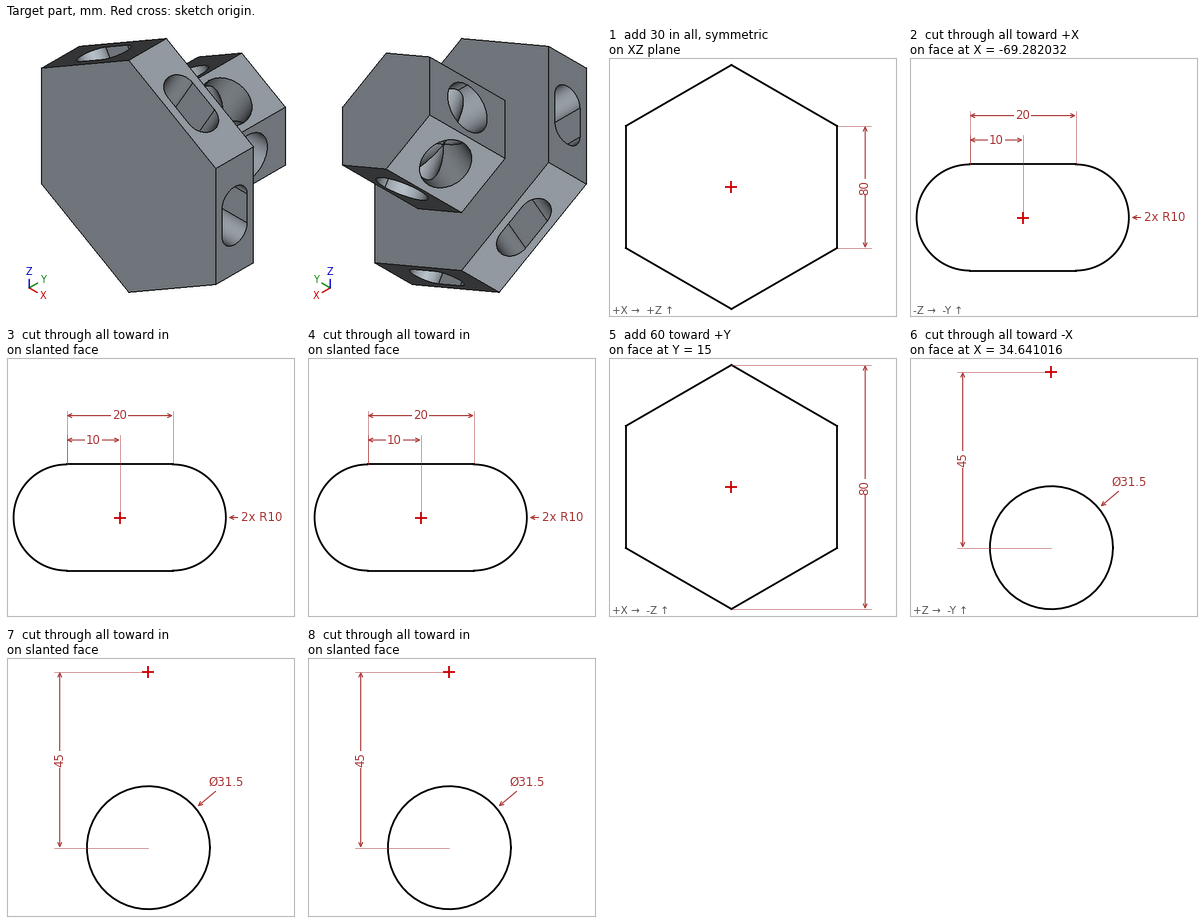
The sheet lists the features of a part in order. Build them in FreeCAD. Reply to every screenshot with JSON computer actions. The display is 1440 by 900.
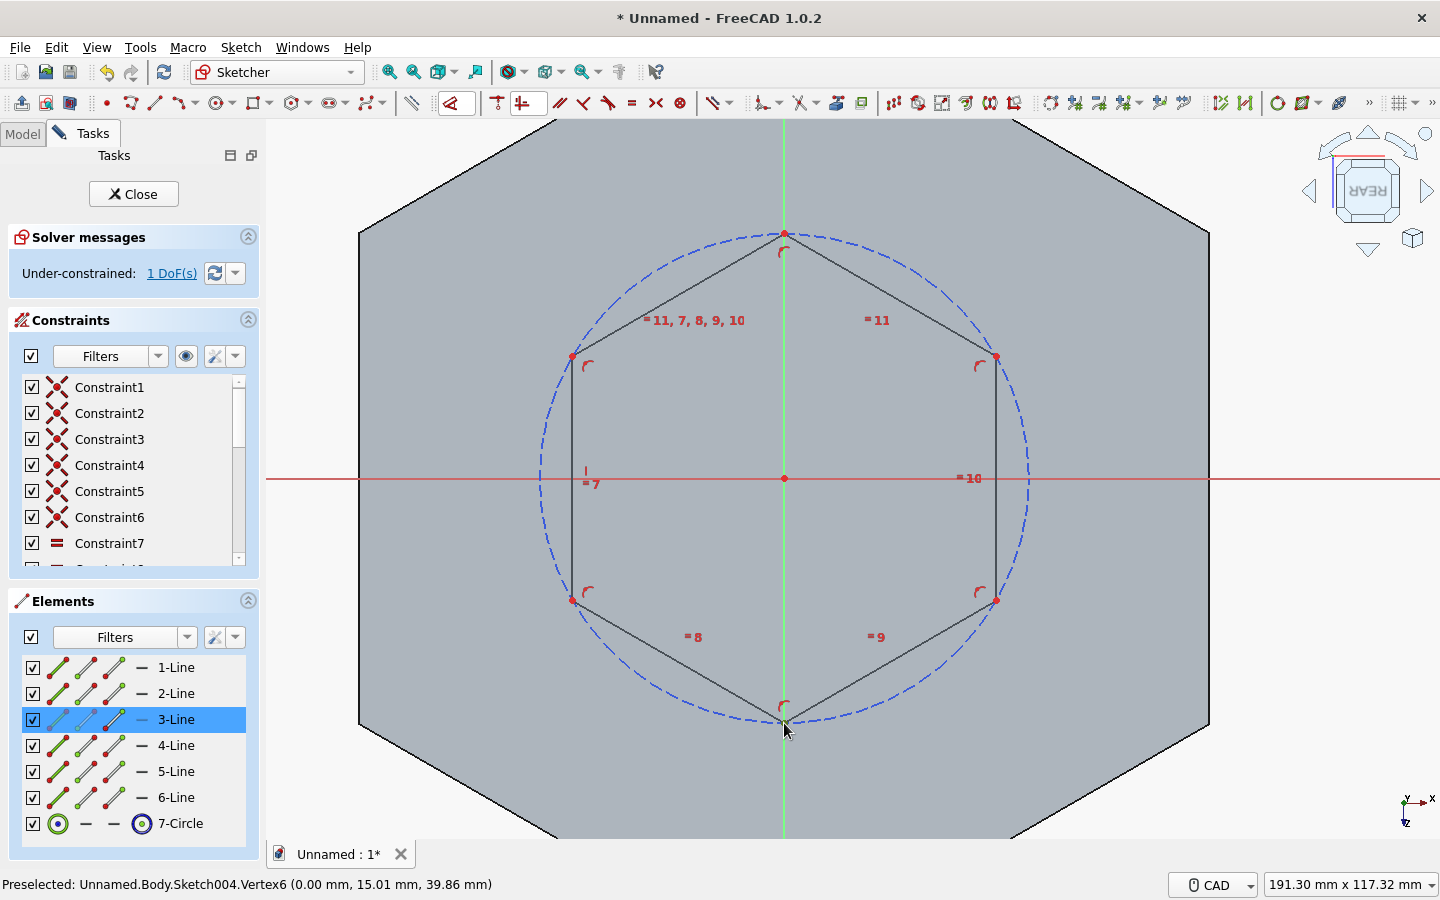
{"action": "left_click", "coordinate": [784, 234]}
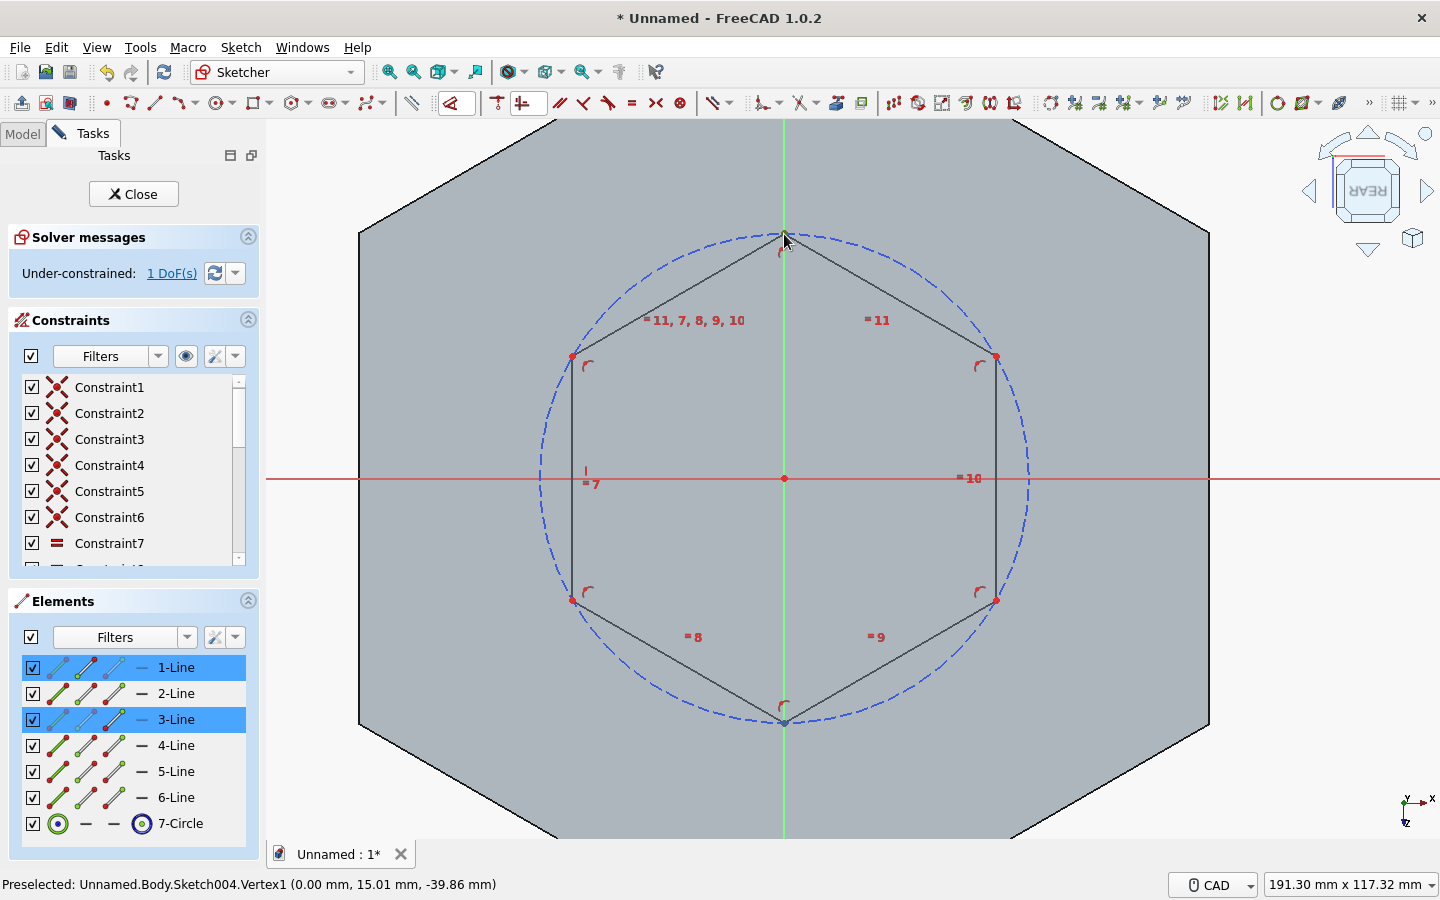
{"action": "key", "text": "i"}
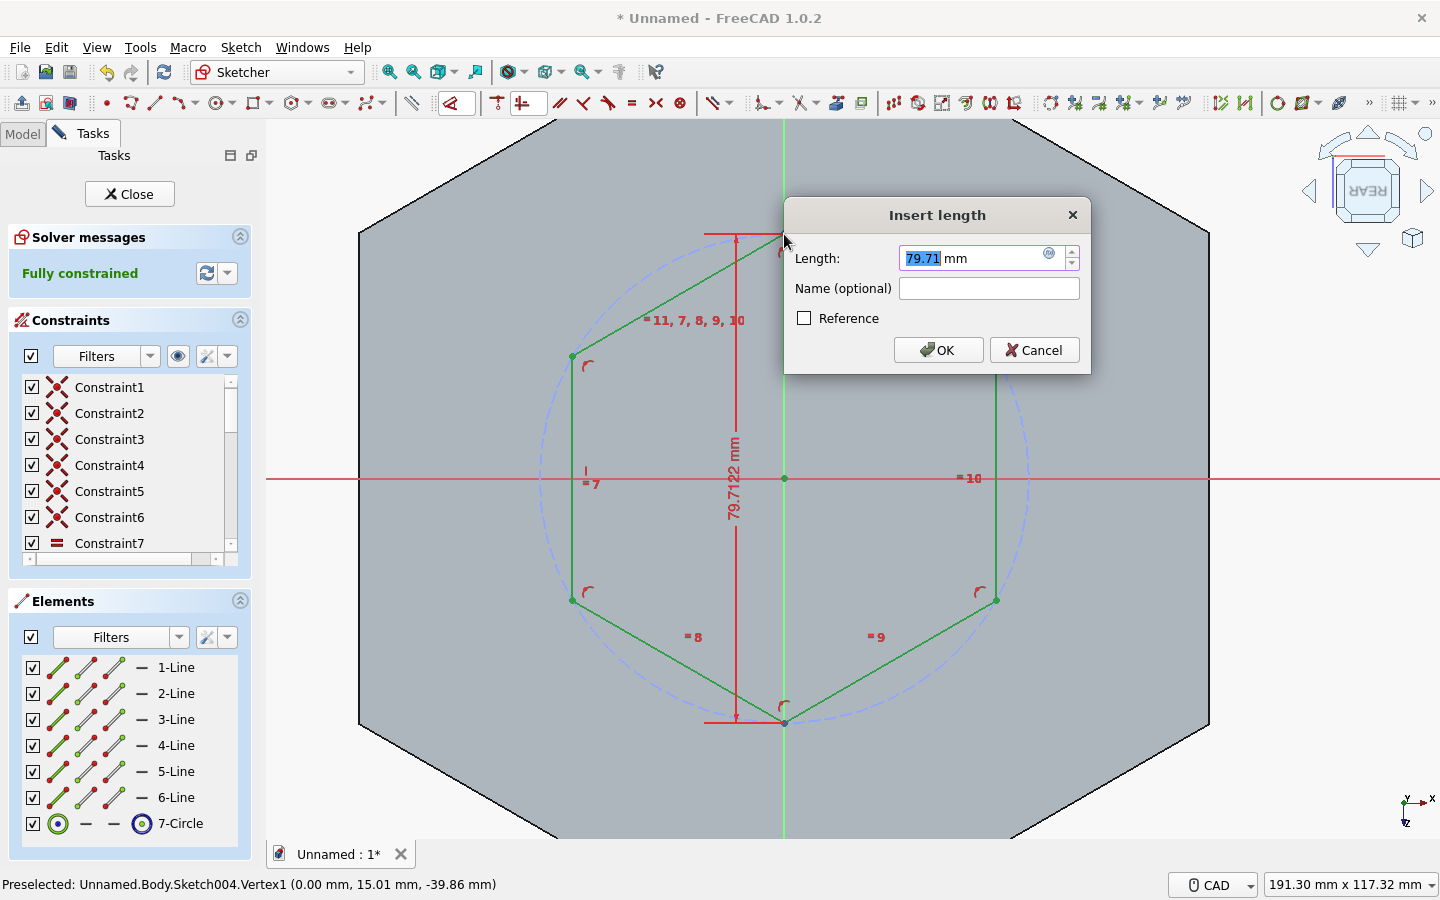
{"action": "type", "text": "80"}
{"action": "key", "text": "Return"}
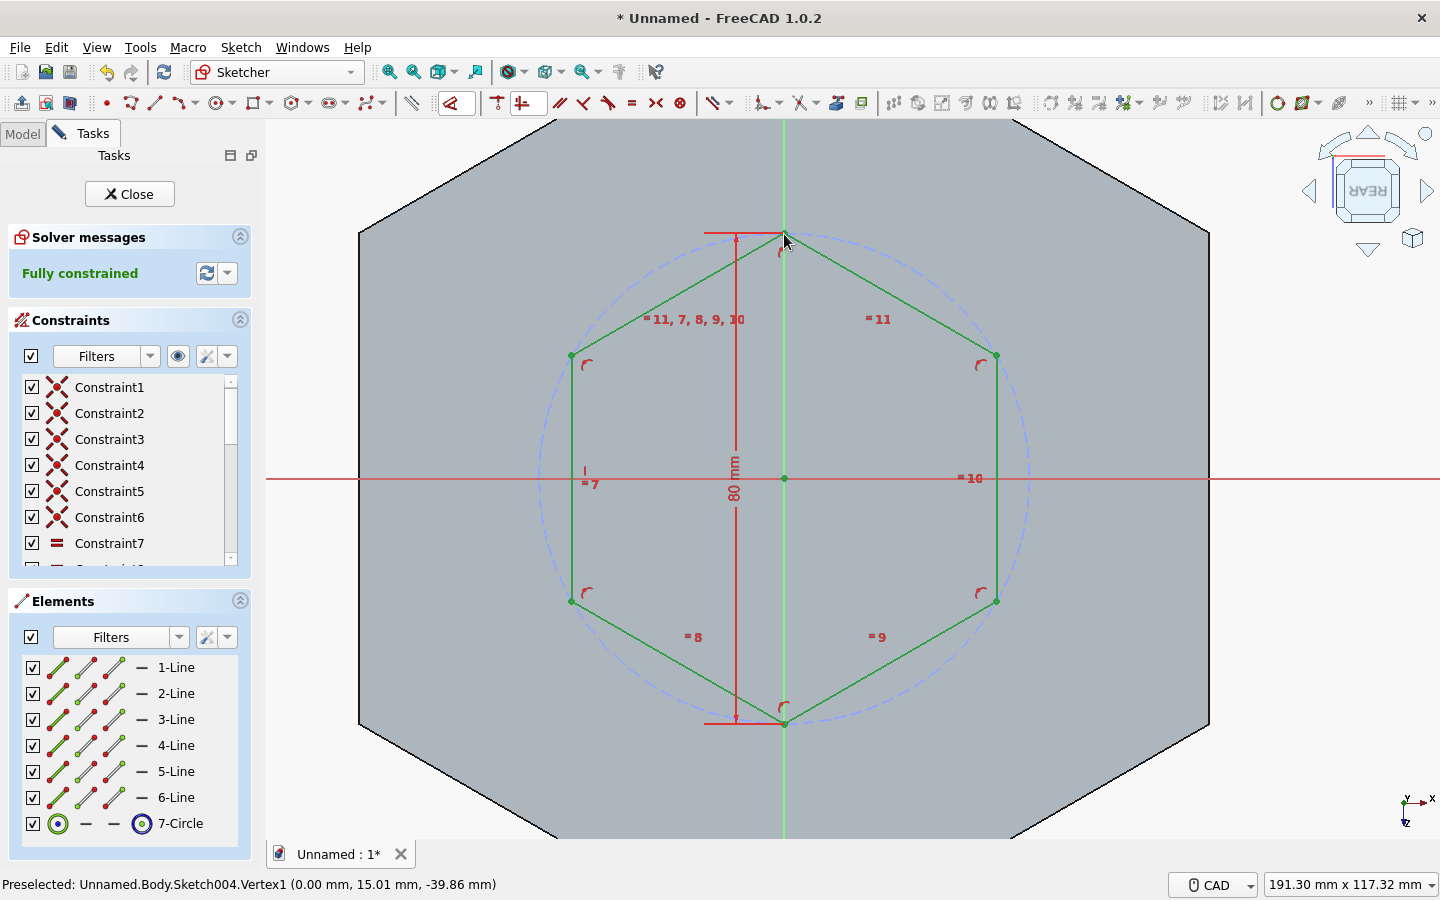
{"action": "left_click", "coordinate": [130, 194]}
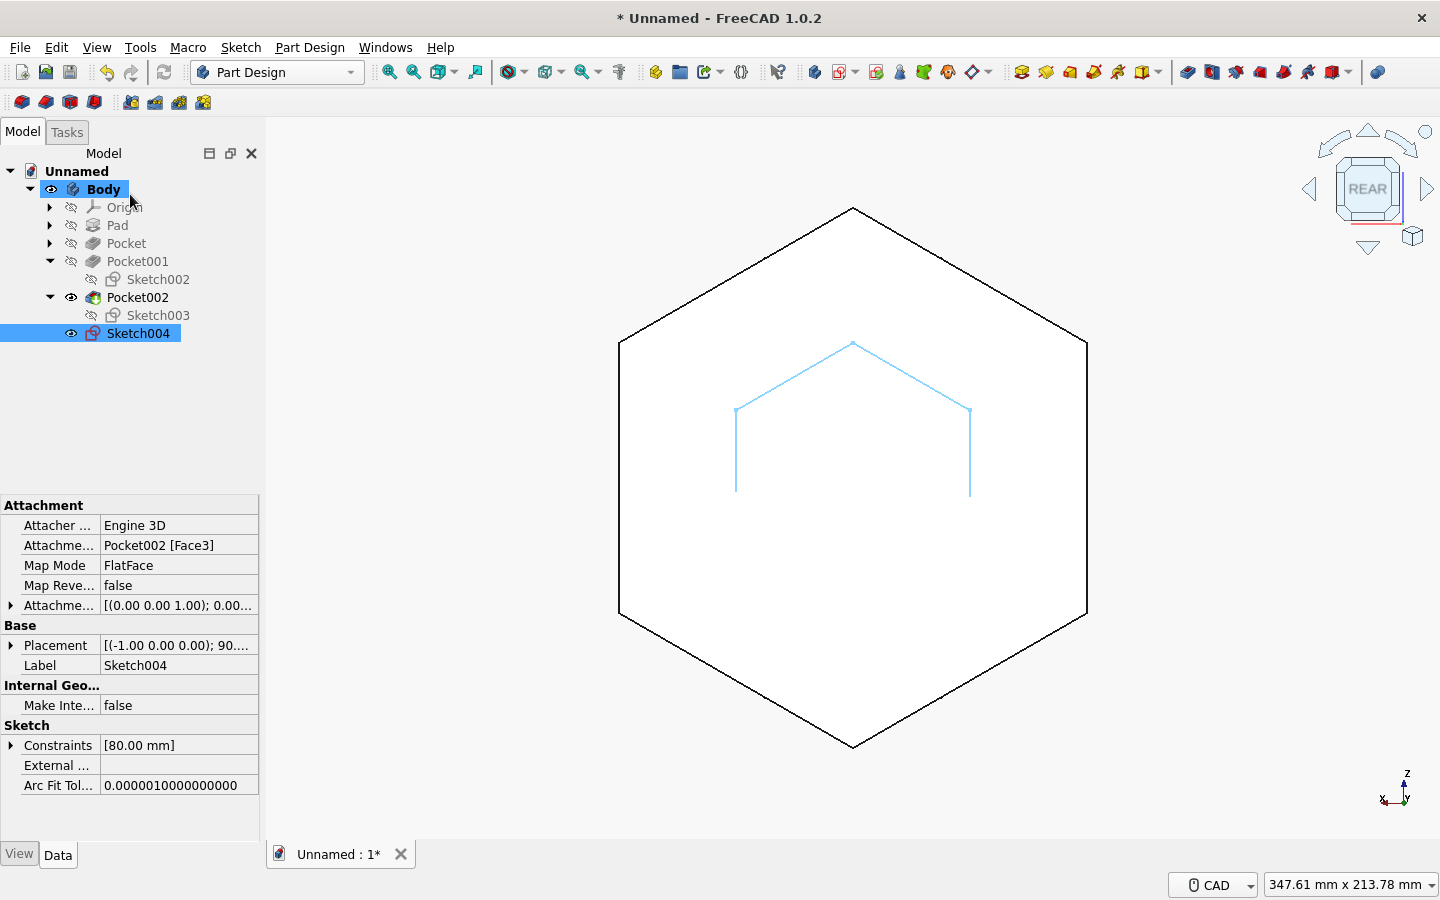
{"action": "left_click", "coordinate": [1022, 72]}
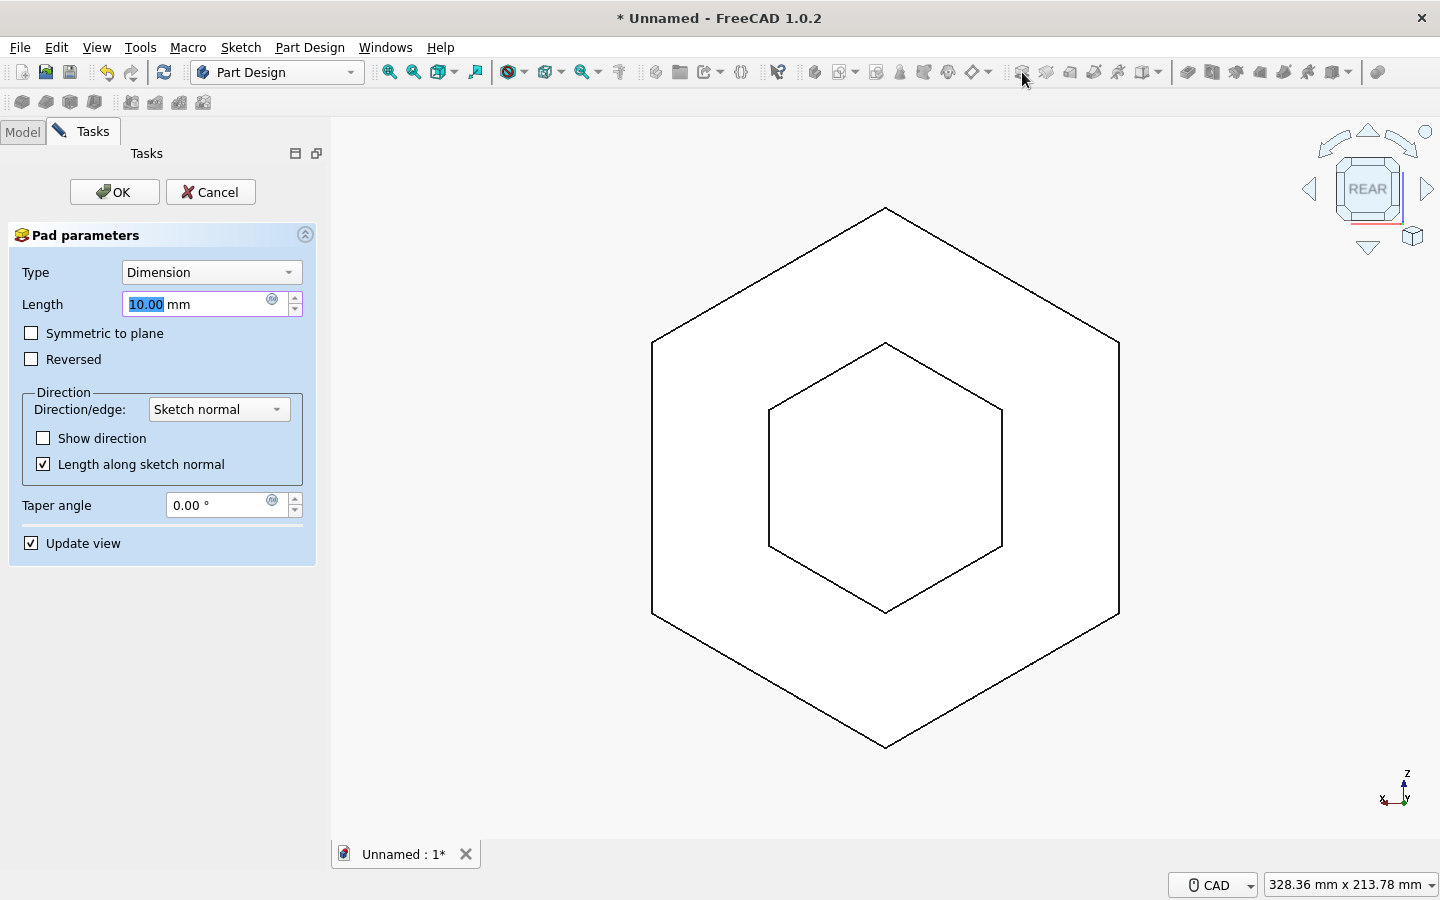
{"action": "type", "text": "60"}
{"action": "key", "text": "Tab"}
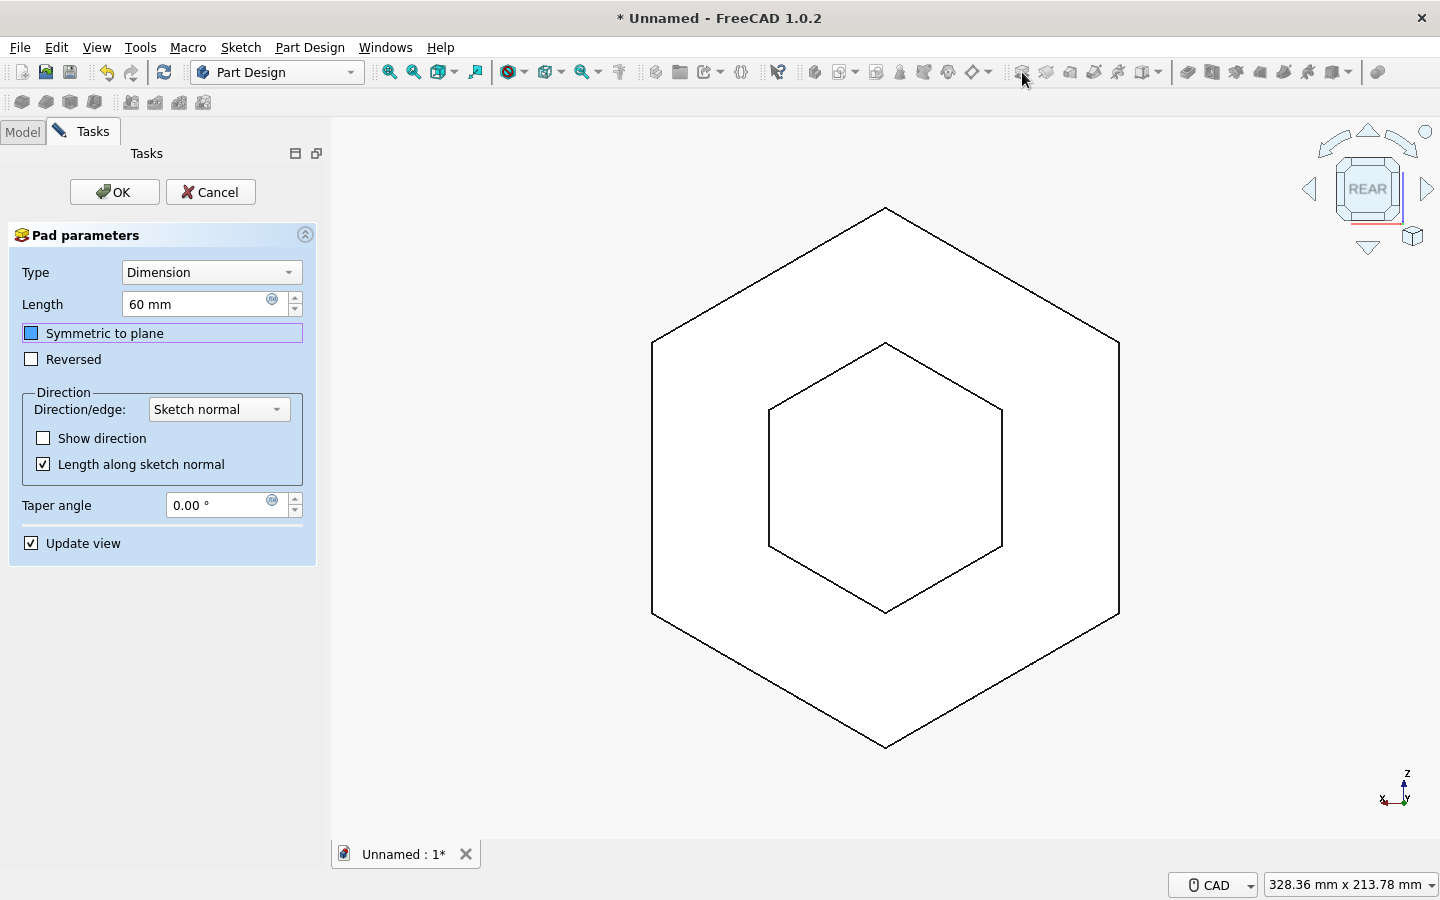
{"action": "left_click", "coordinate": [115, 192]}